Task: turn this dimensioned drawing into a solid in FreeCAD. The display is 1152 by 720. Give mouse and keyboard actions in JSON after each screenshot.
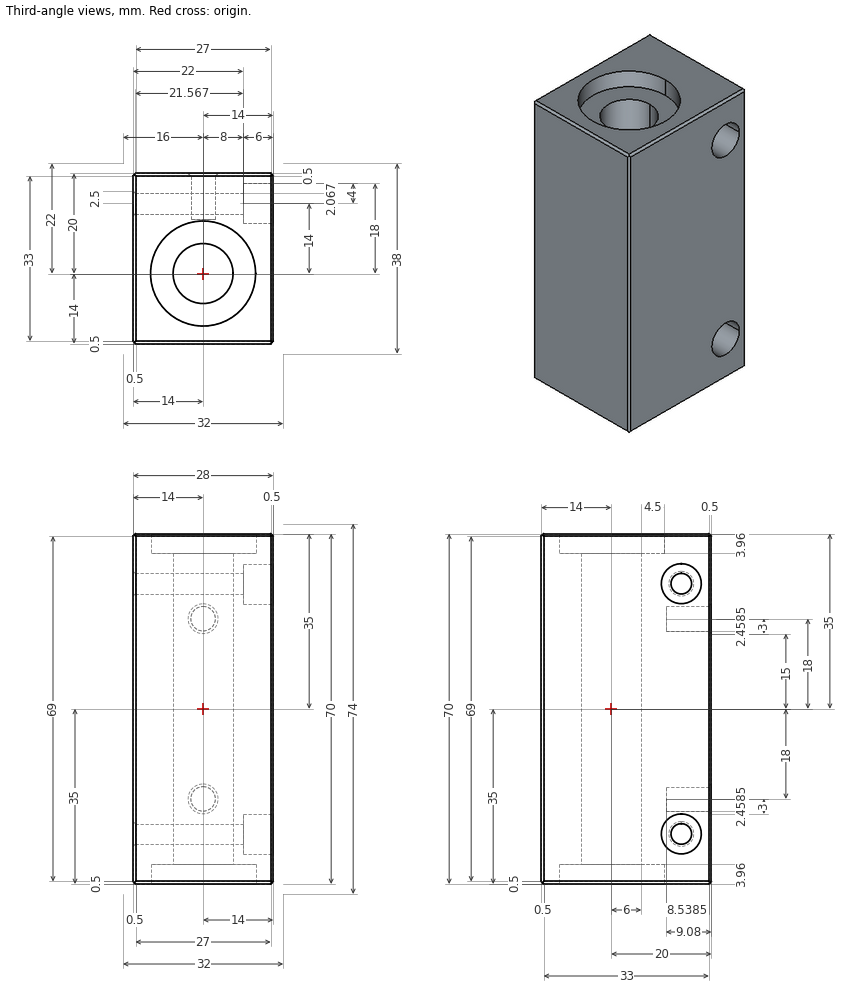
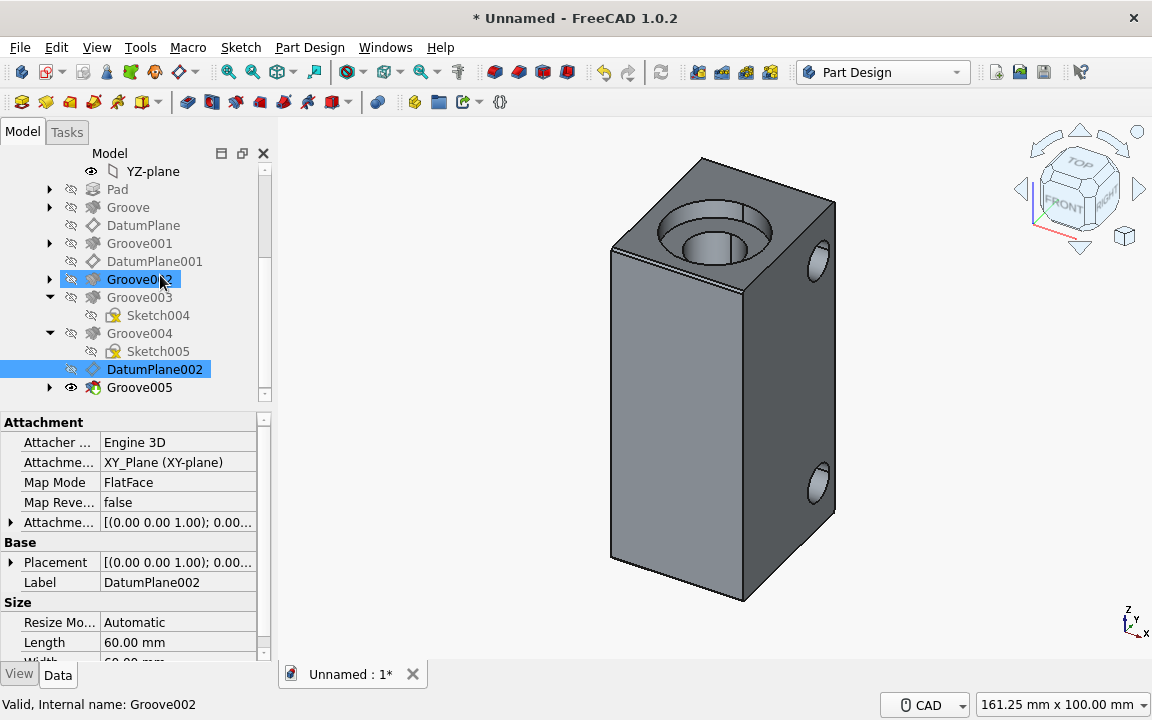
{"action": "scroll", "coordinate": [160, 275], "scroll_direction": "up", "scroll_amount": 15}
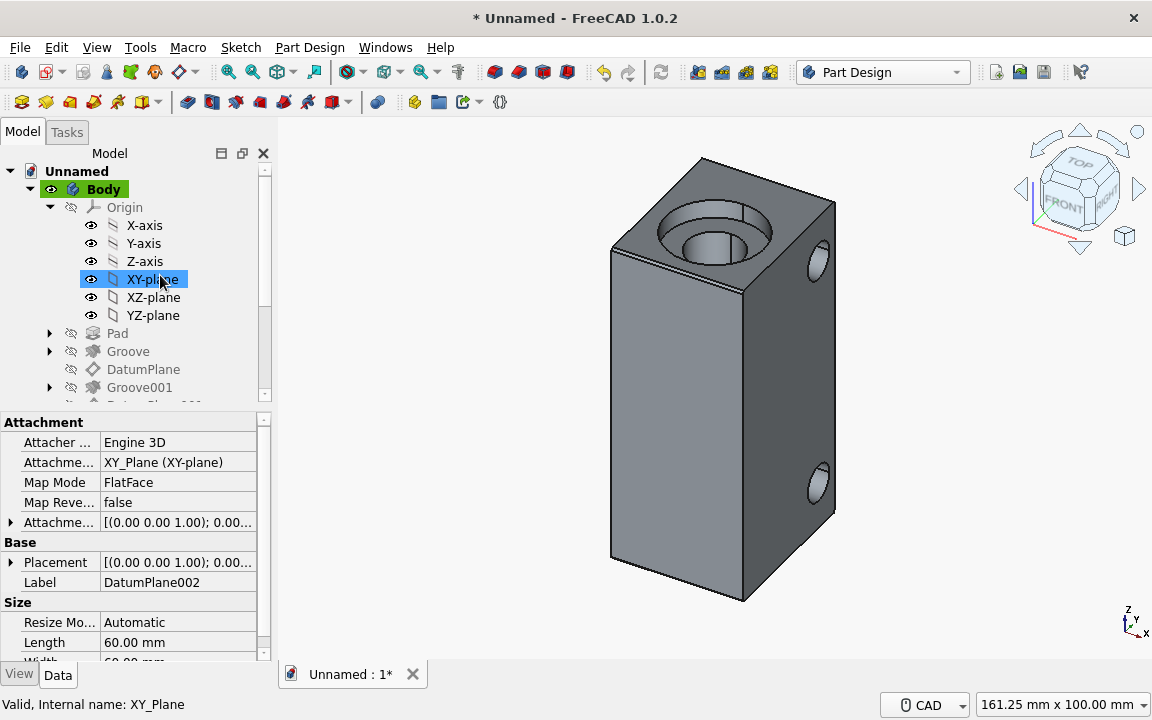
{"action": "left_click", "coordinate": [136, 279]}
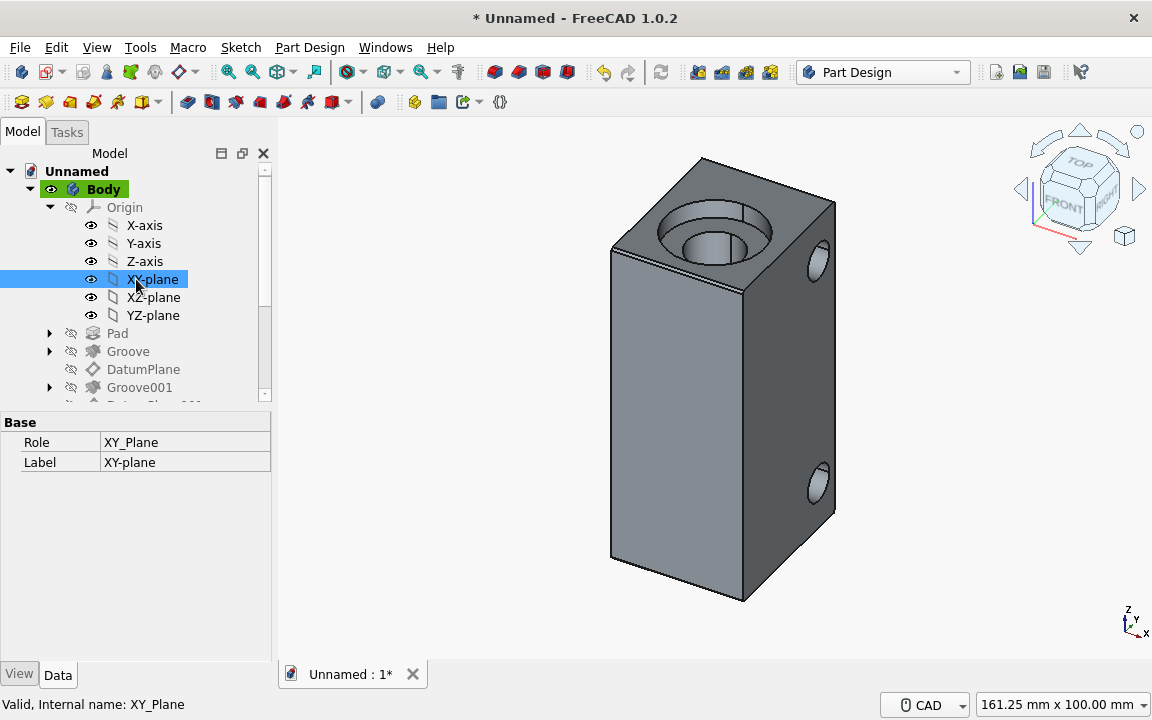
{"action": "left_click", "coordinate": [180, 72]}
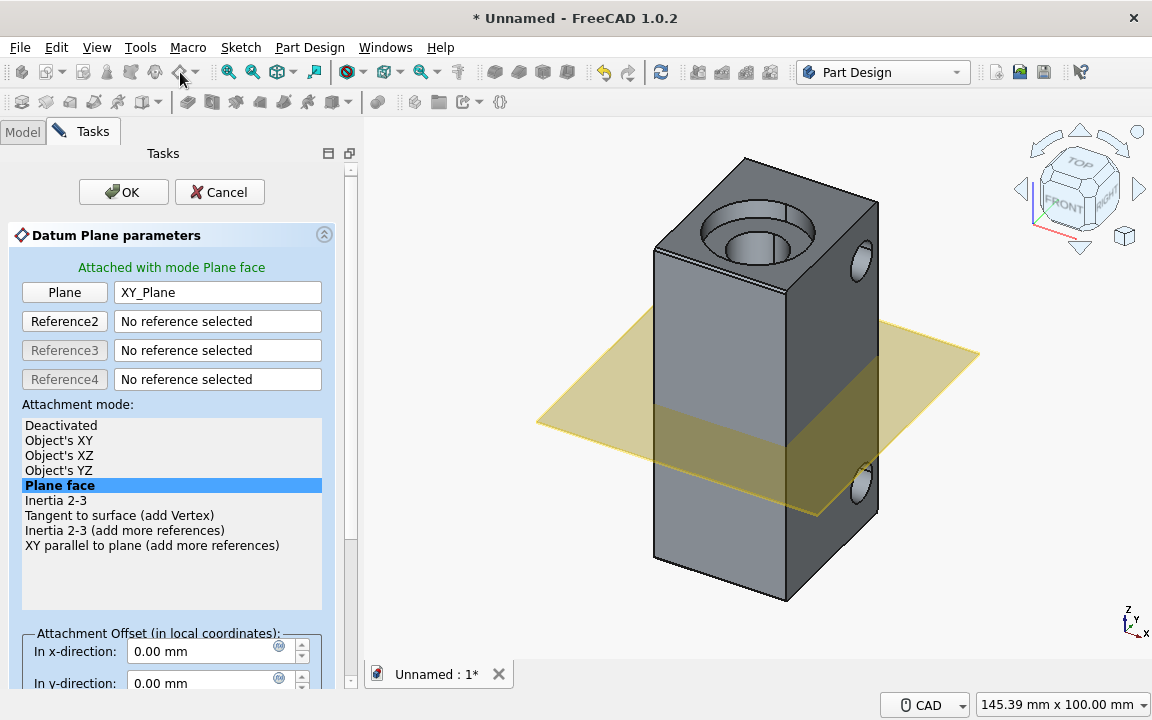
{"action": "scroll", "coordinate": [351, 426], "scroll_direction": "down", "scroll_amount": 2}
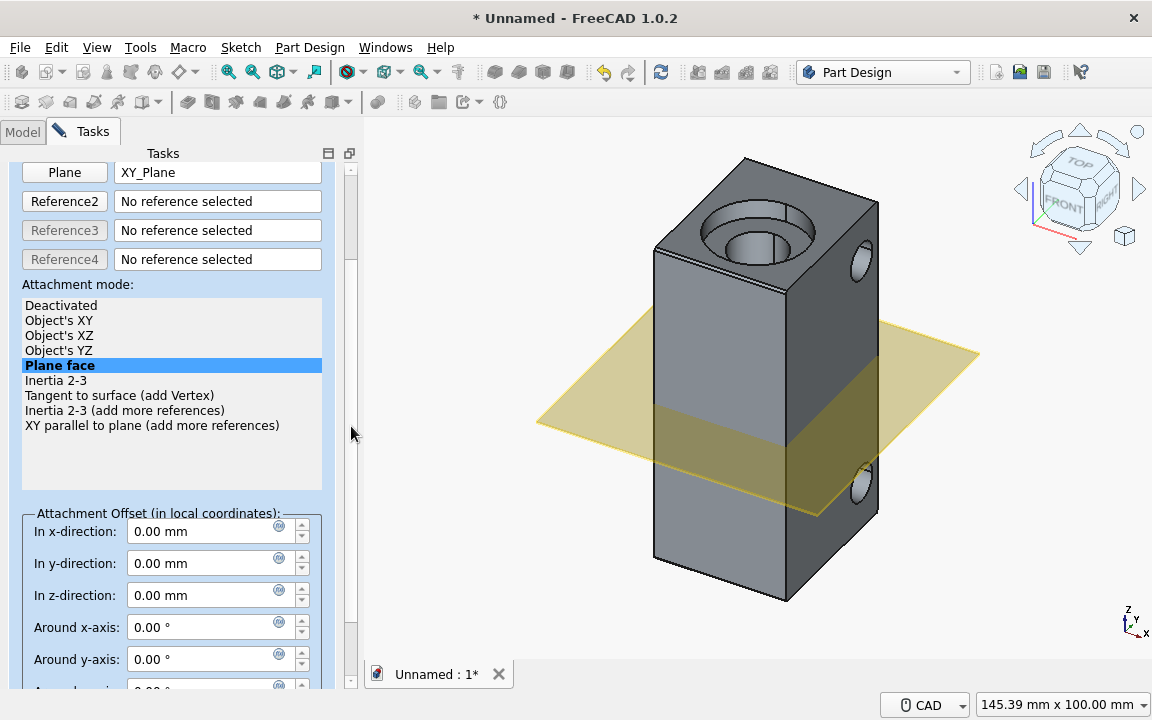
{"action": "triple_click", "coordinate": [210, 595]}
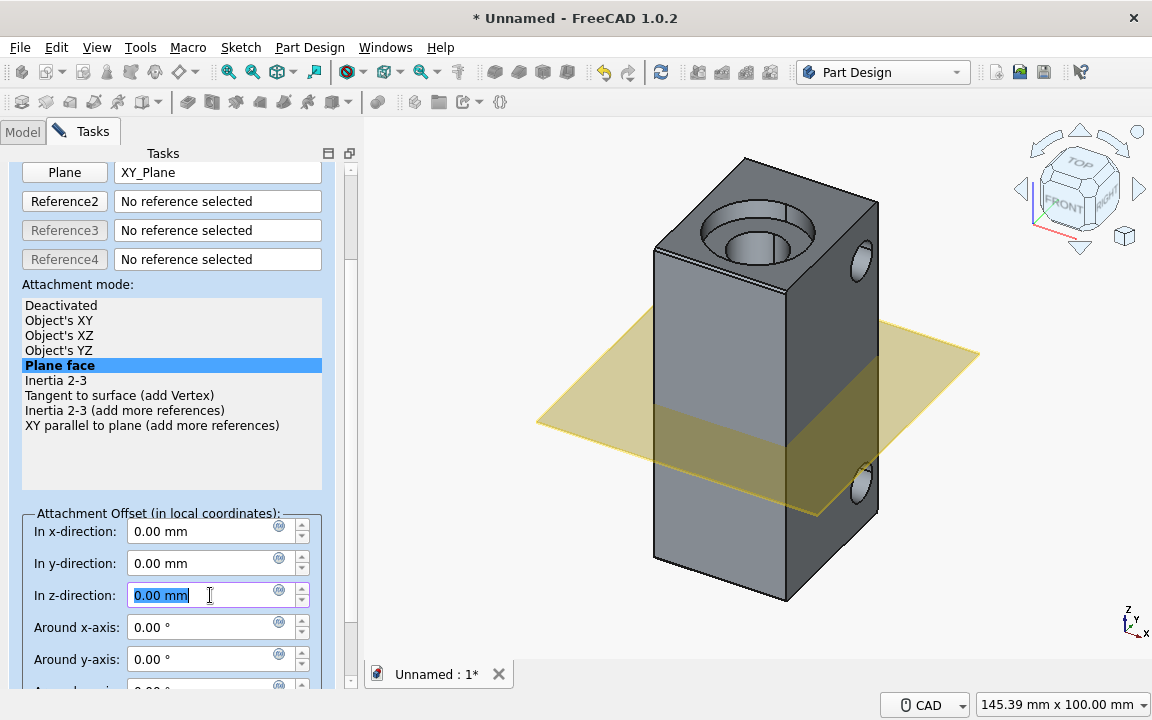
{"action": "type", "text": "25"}
{"action": "key", "text": "Tab"}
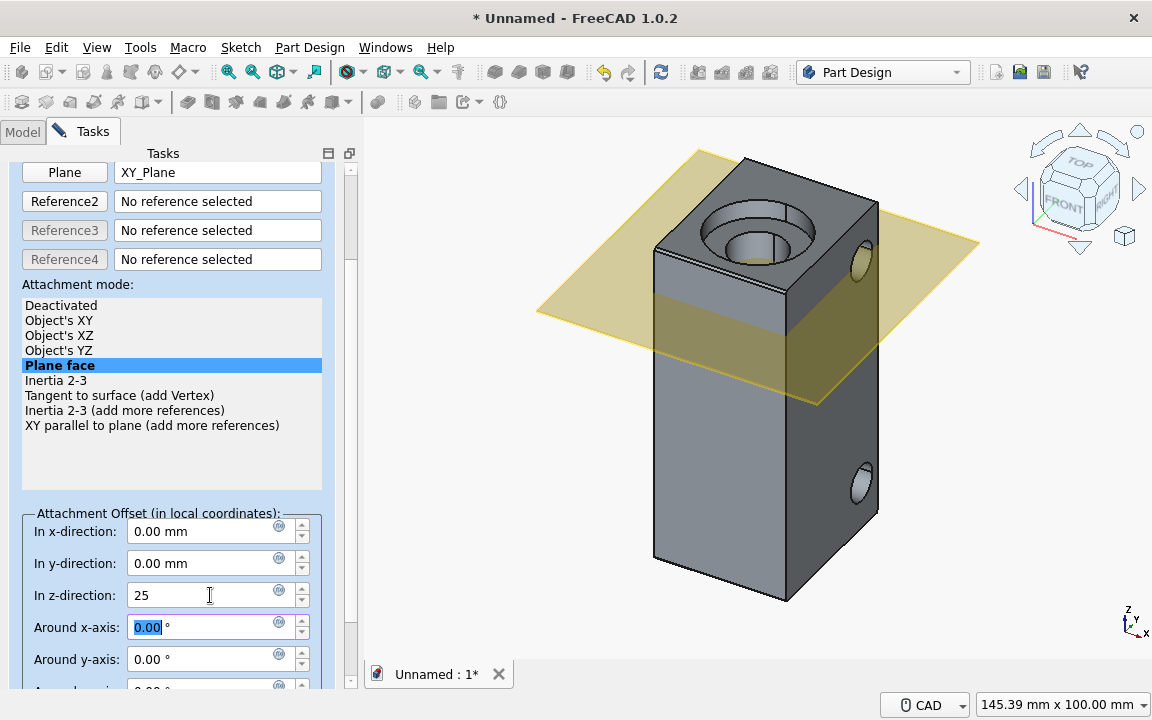
{"action": "scroll", "coordinate": [351, 426], "scroll_direction": "up", "scroll_amount": 3}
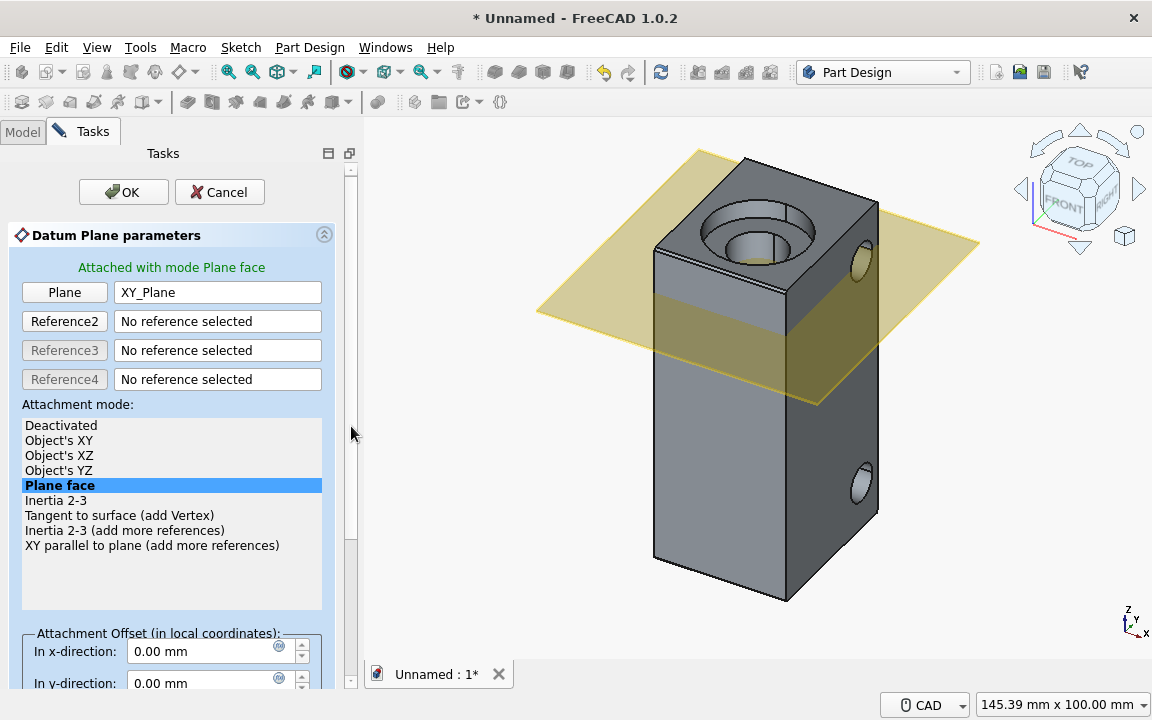
{"action": "left_click", "coordinate": [124, 192]}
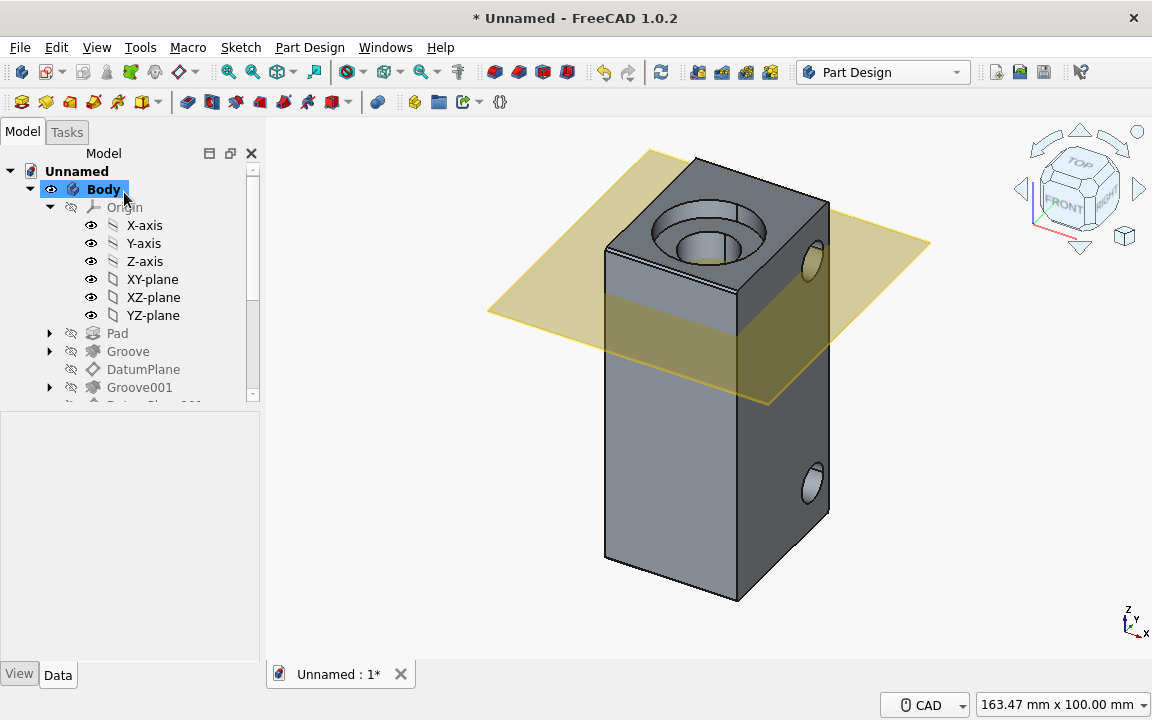
{"action": "scroll", "coordinate": [100, 275], "scroll_direction": "down", "scroll_amount": 3}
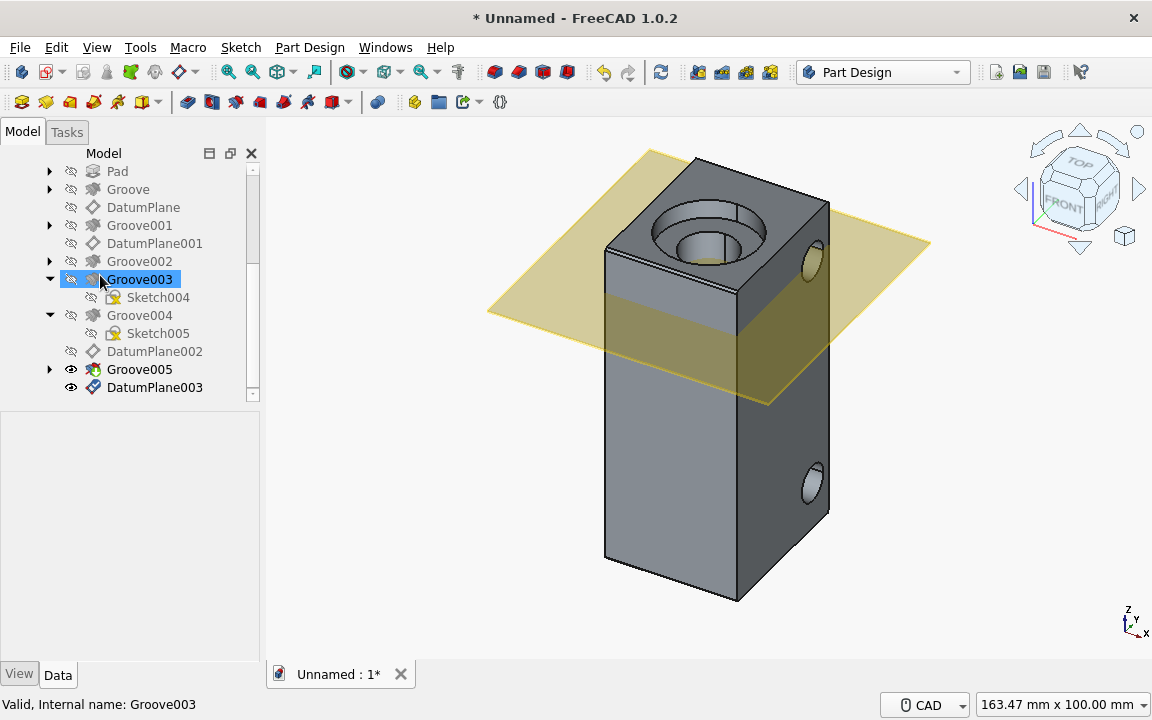
{"action": "left_click", "coordinate": [116, 387]}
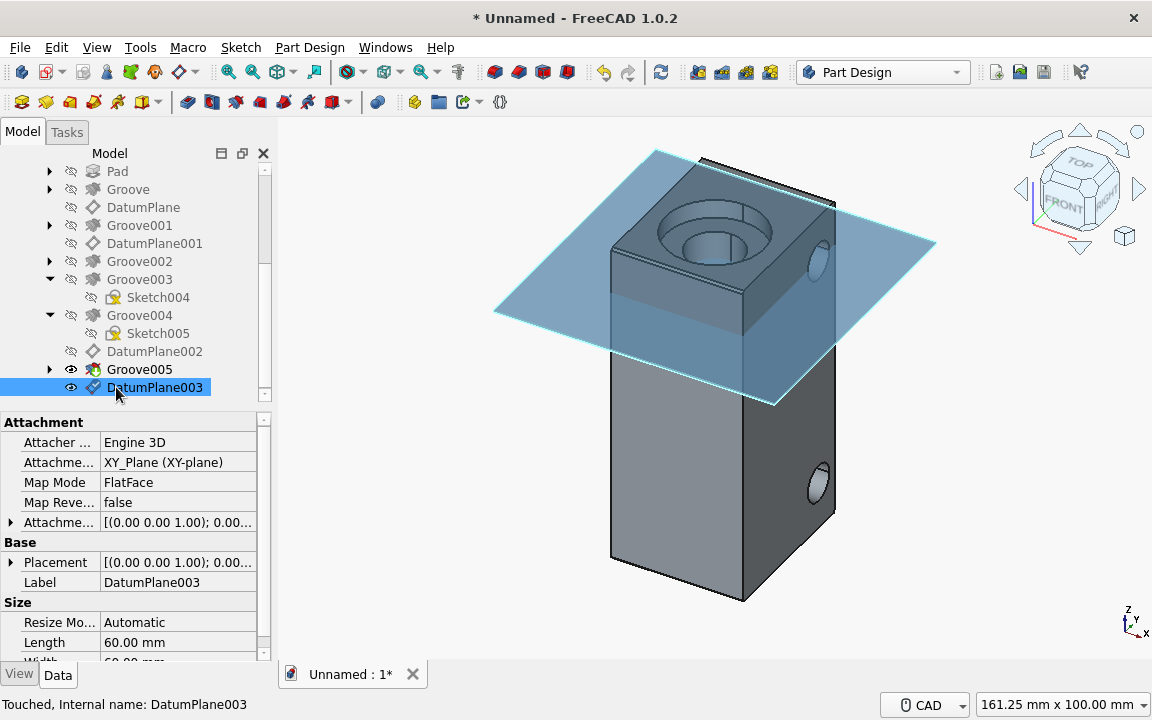
{"action": "left_click", "coordinate": [46, 72]}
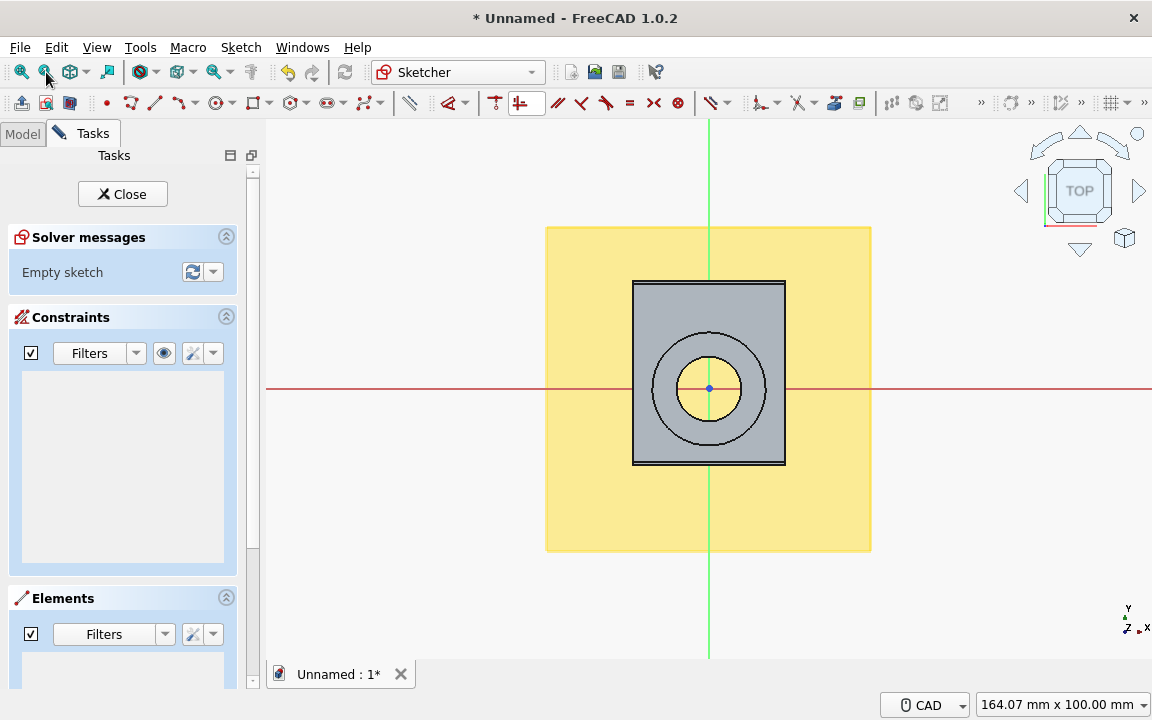
{"action": "left_click", "coordinate": [70, 104]}